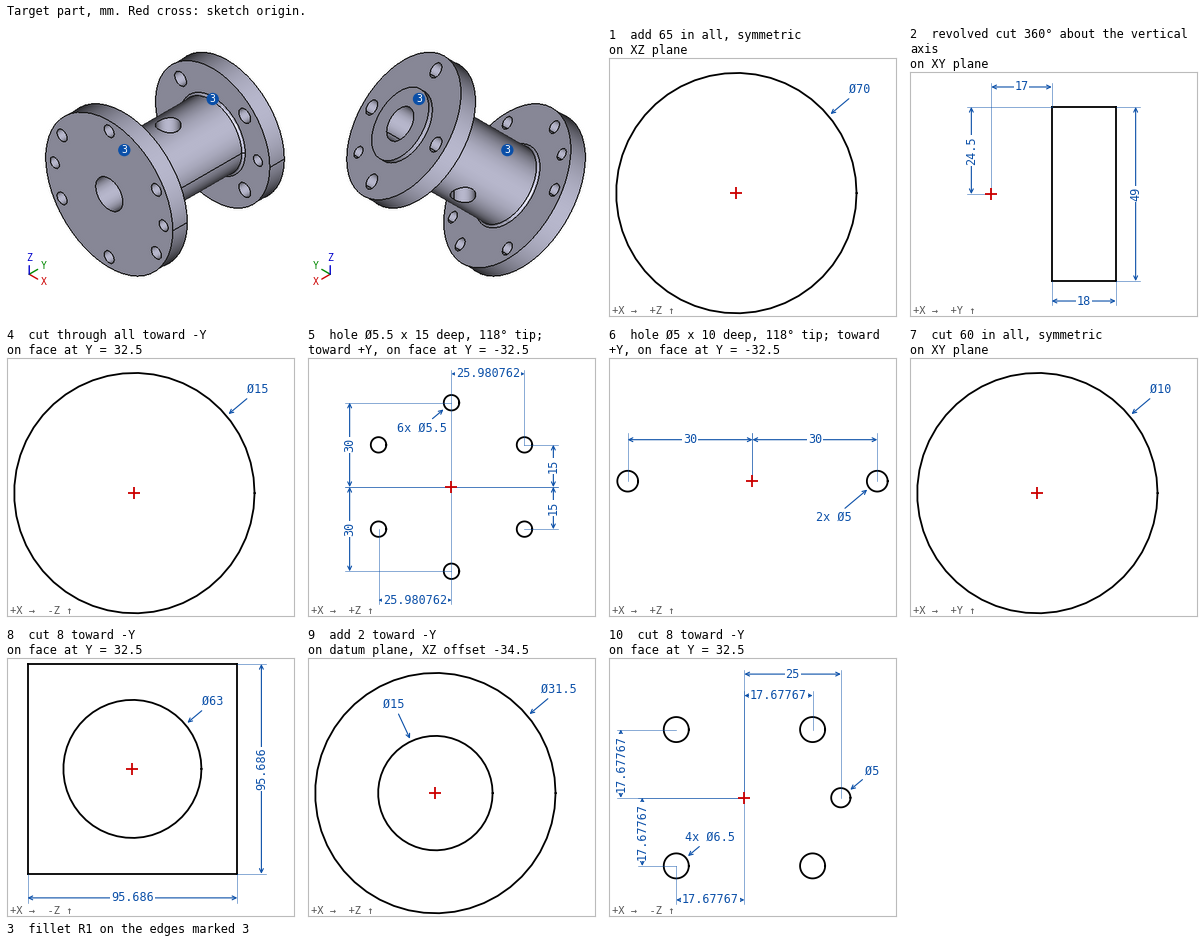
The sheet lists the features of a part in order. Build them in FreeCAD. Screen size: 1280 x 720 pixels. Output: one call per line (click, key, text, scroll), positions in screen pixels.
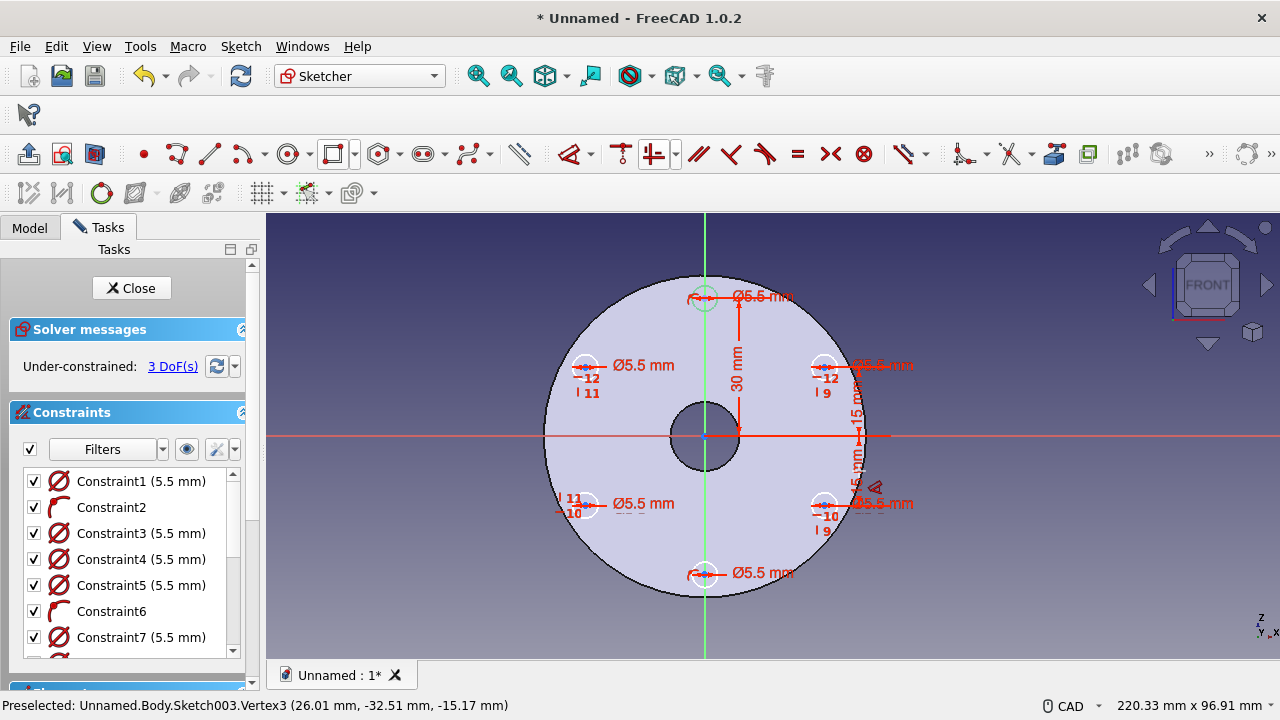
click(705, 575)
click(739, 506)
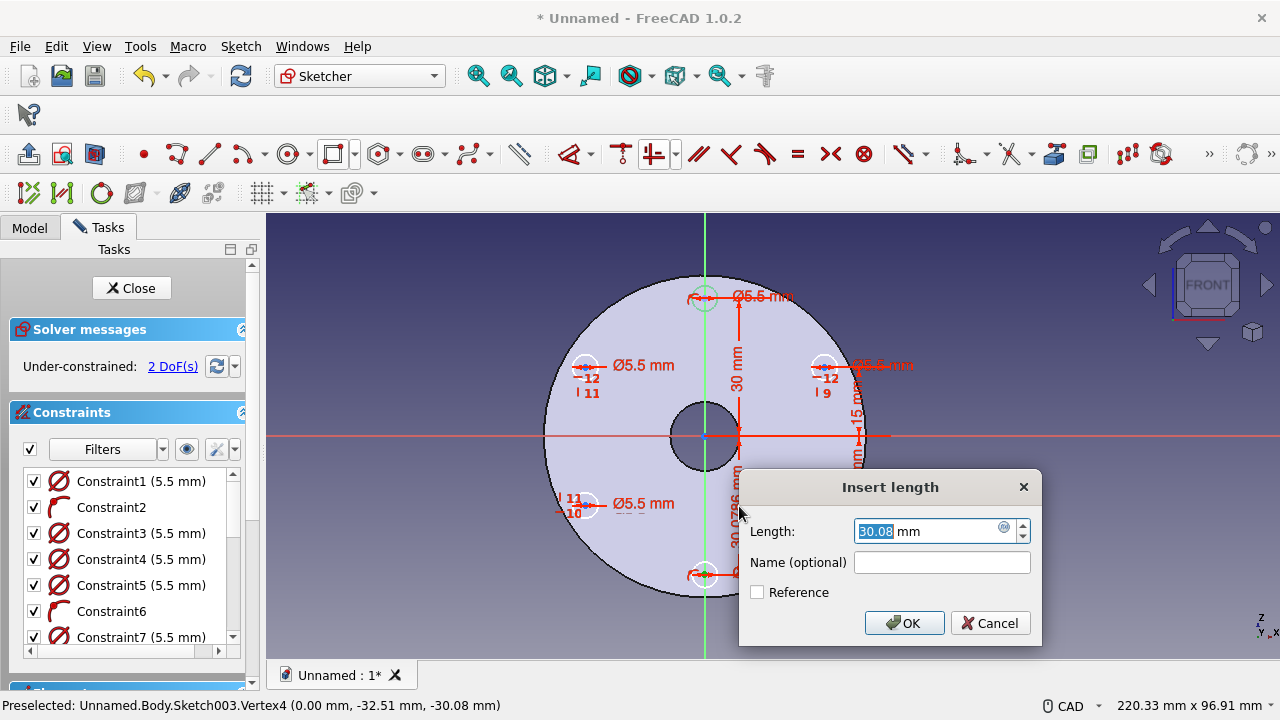
text(30)
key(Return)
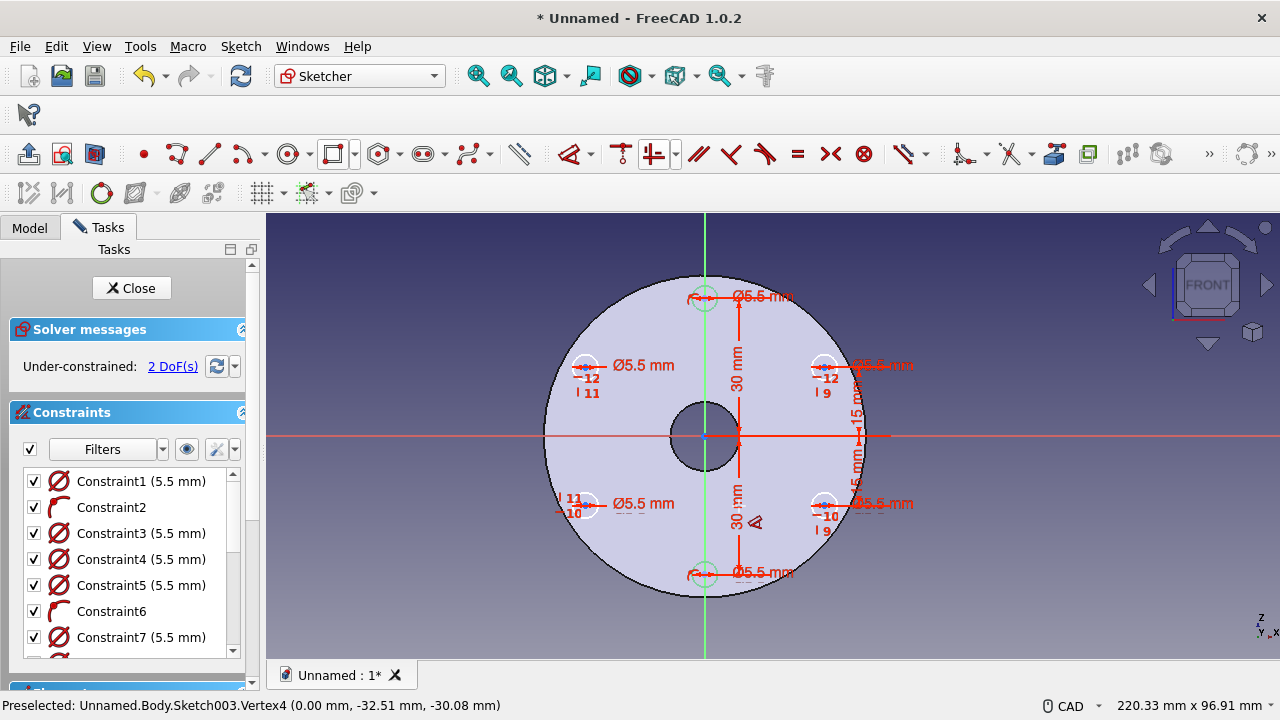
click(825, 367)
click(765, 333)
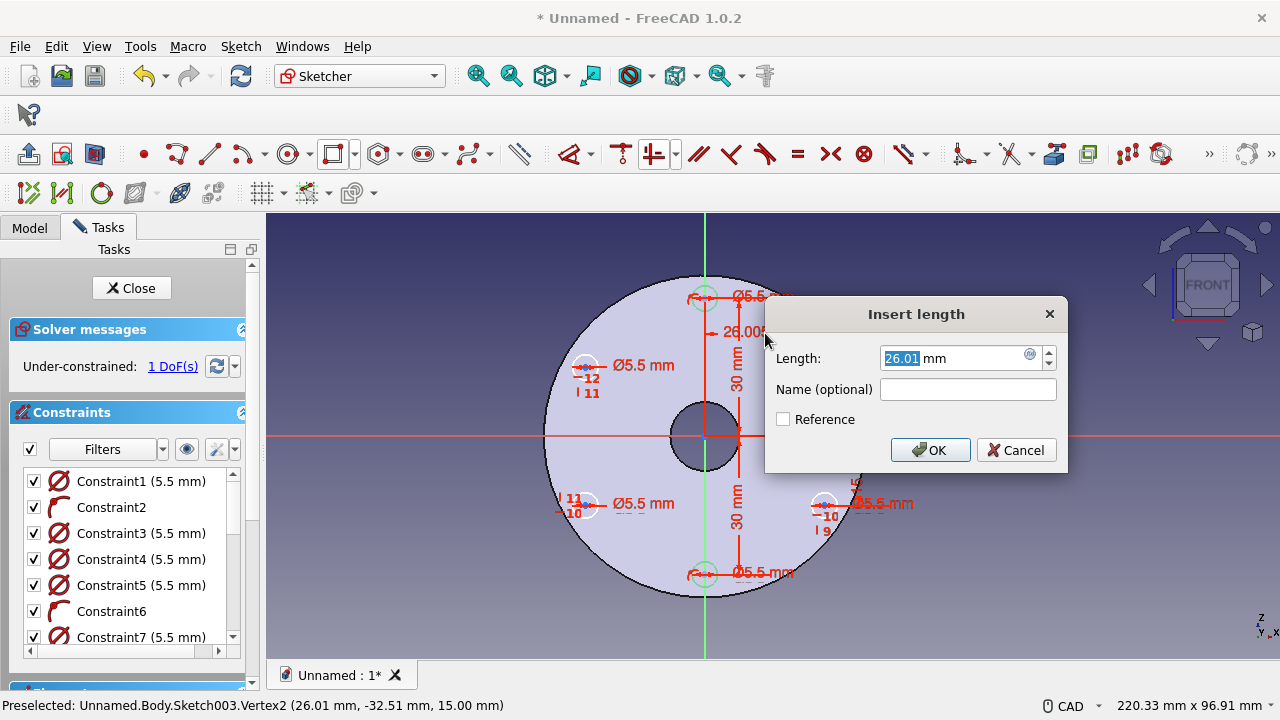
text(25.980762)
key(Return)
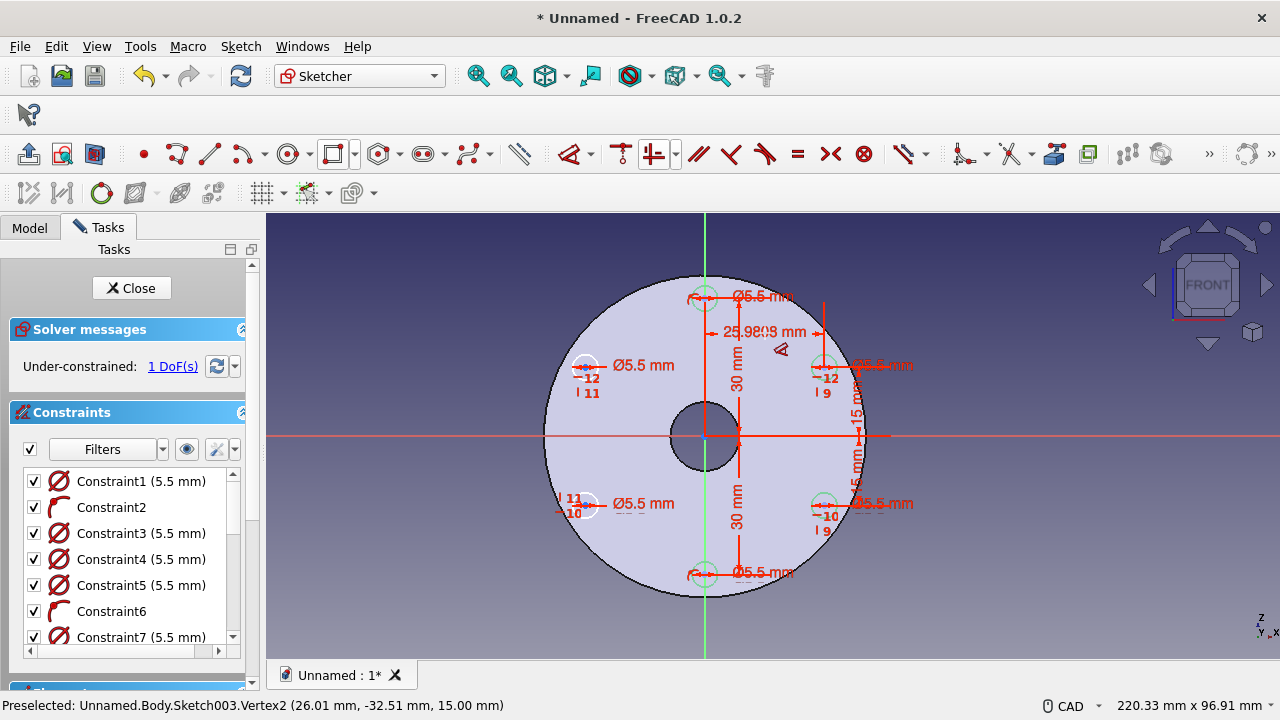
click(585, 506)
click(645, 540)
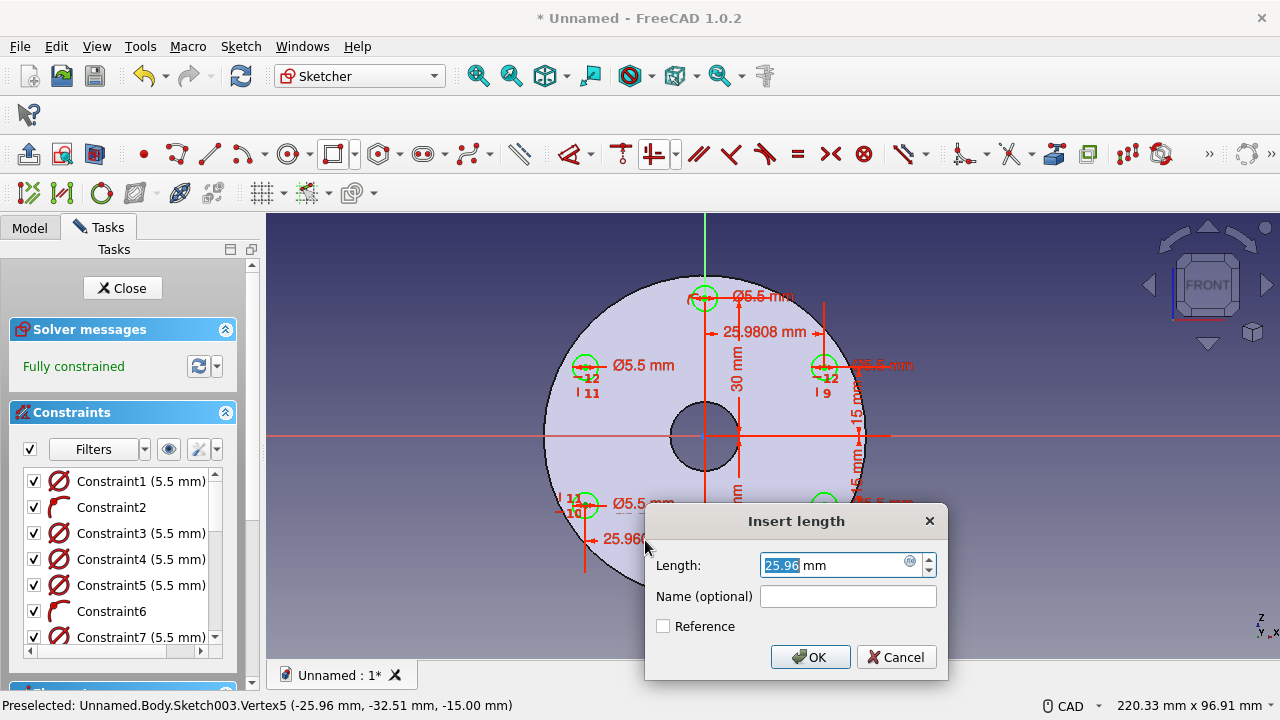
text(25.980762)
key(Return)
key(Escape)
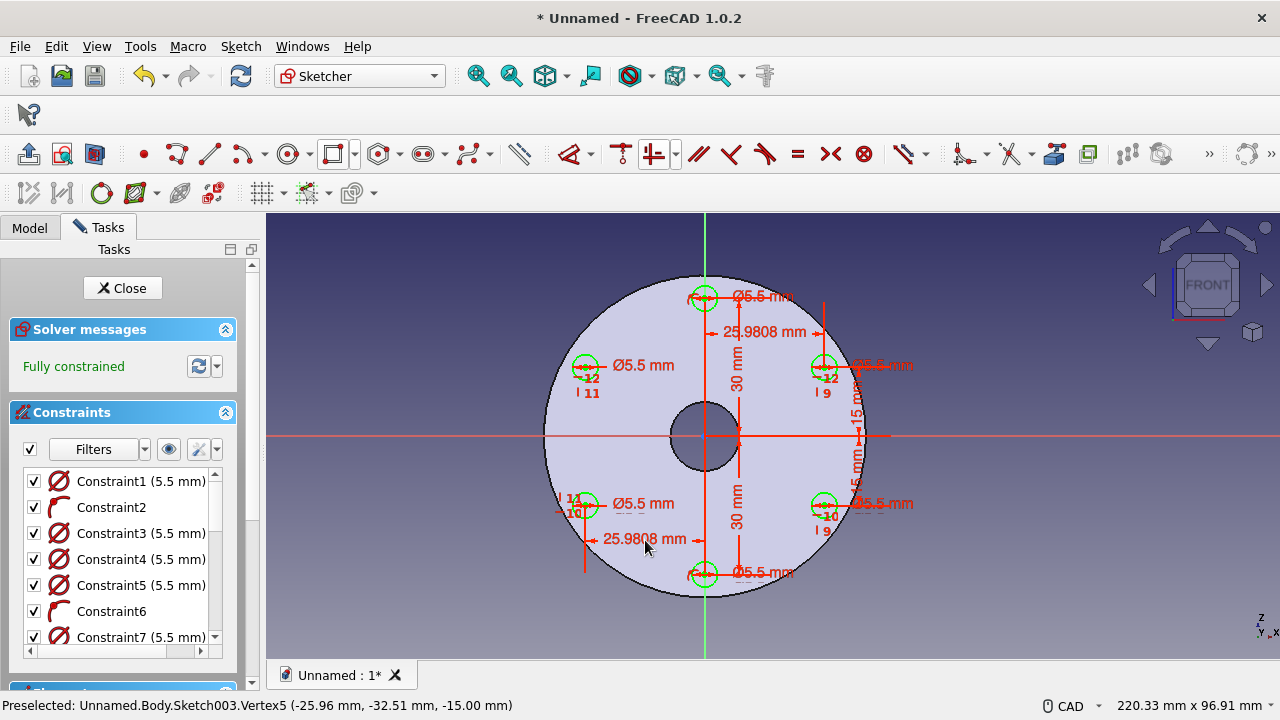
click(123, 288)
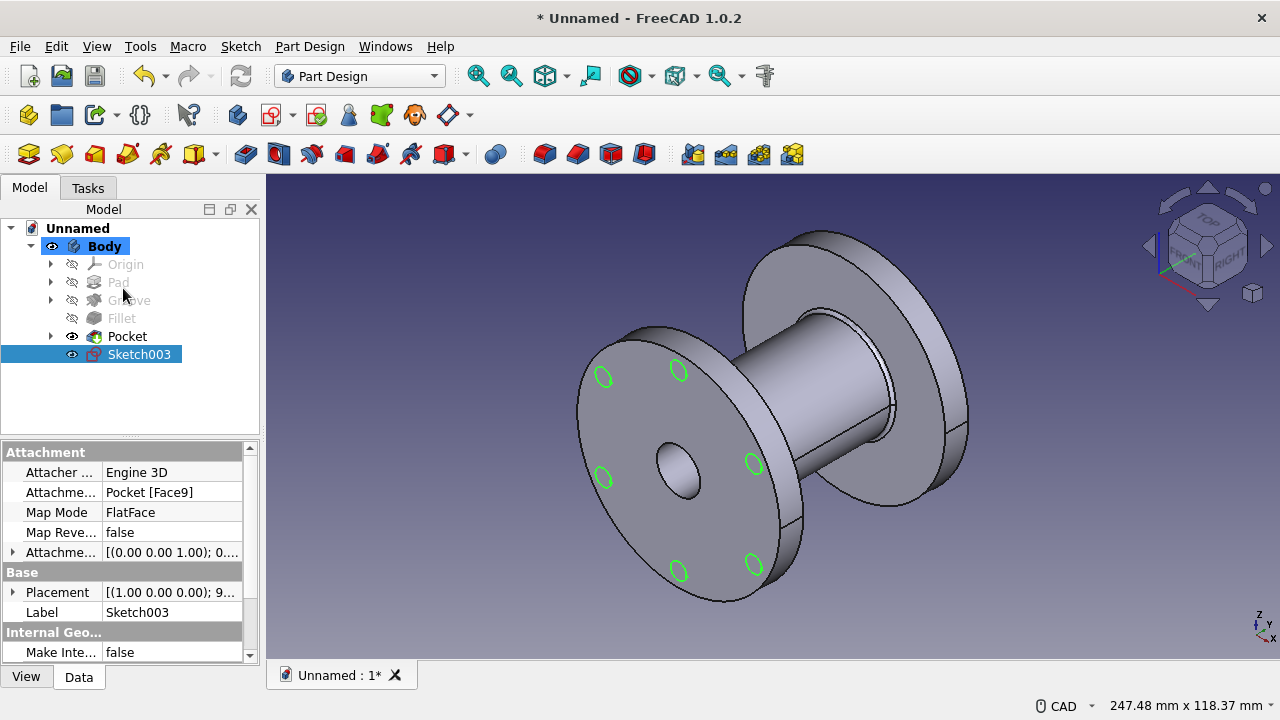
click(279, 154)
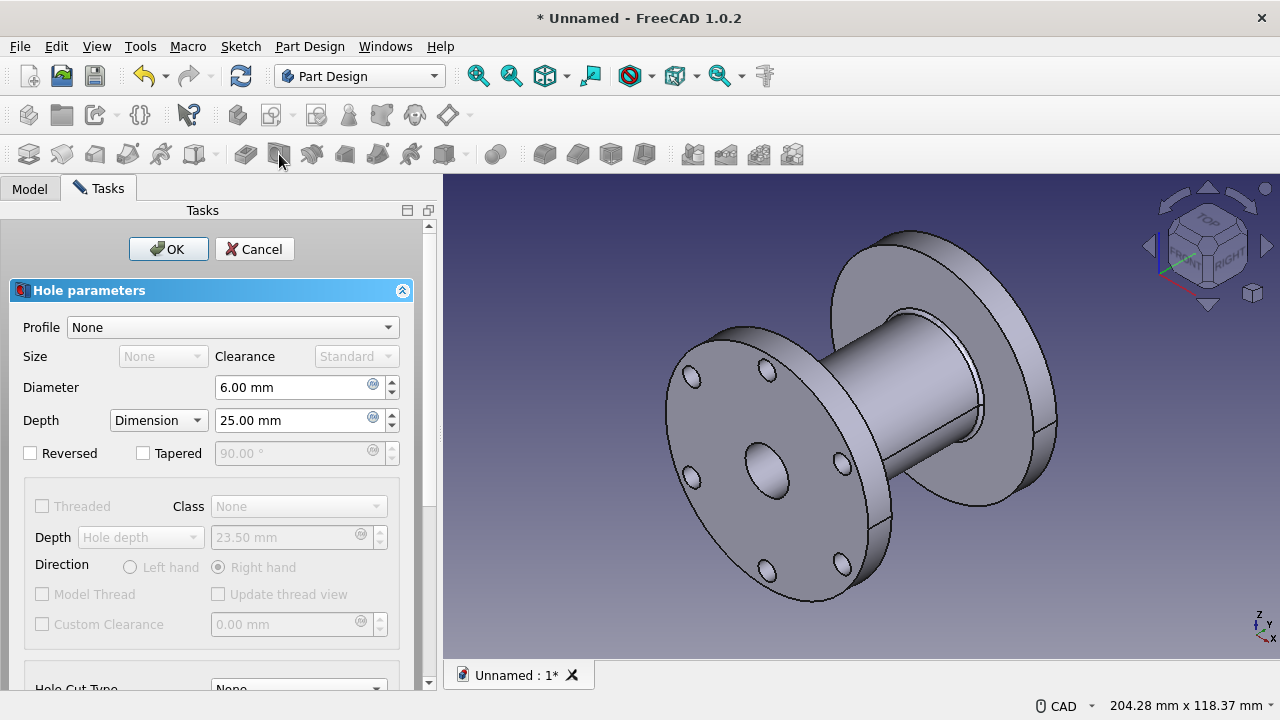
triple_click(300, 388)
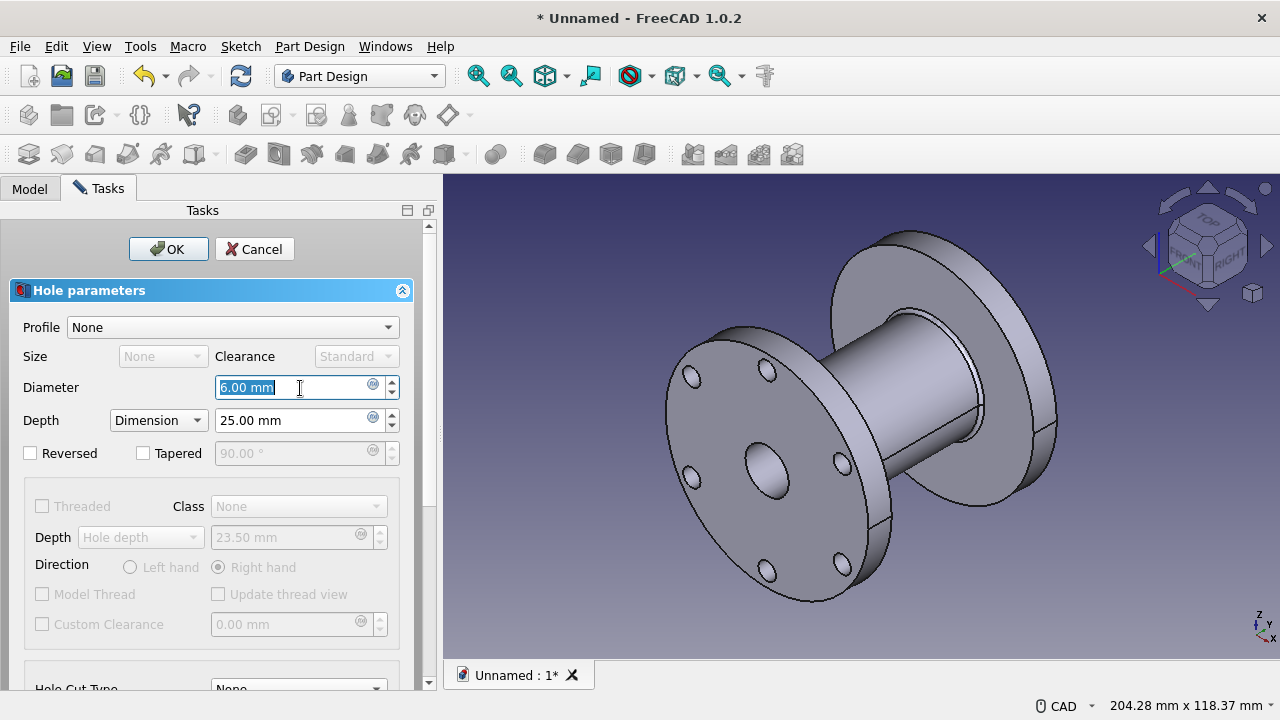
text(5.5)
key(Tab)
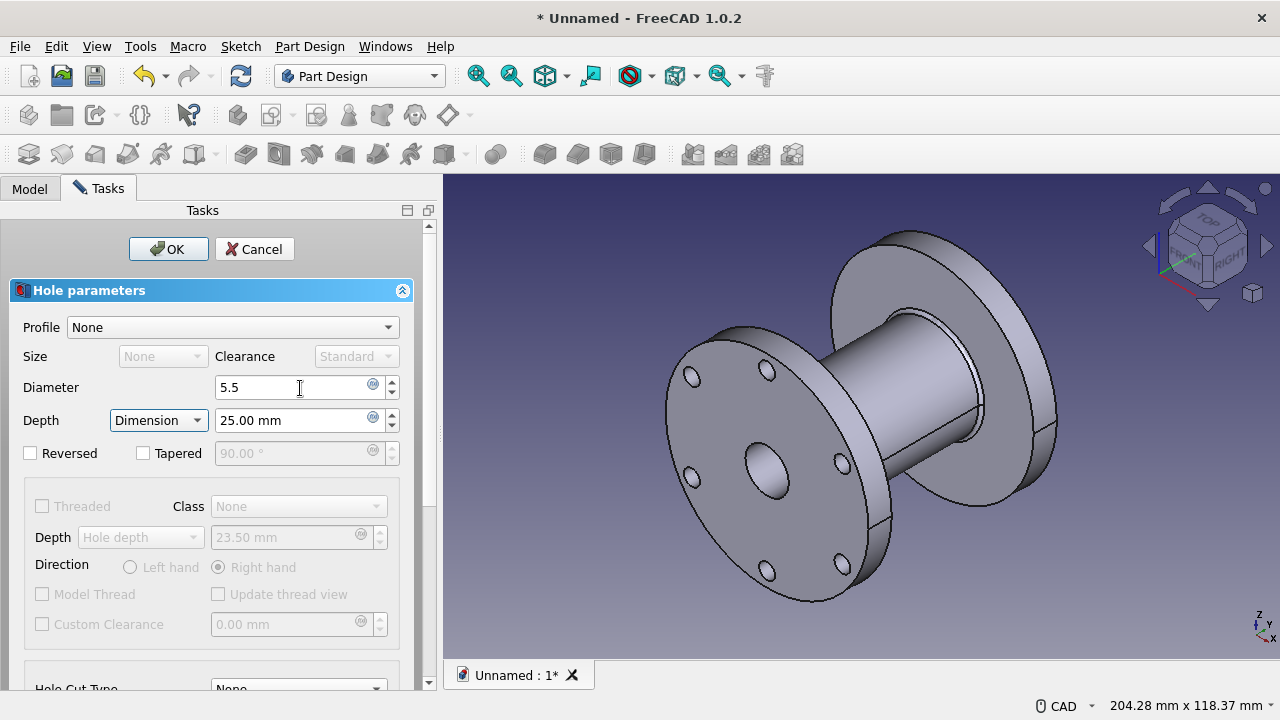
triple_click(300, 420)